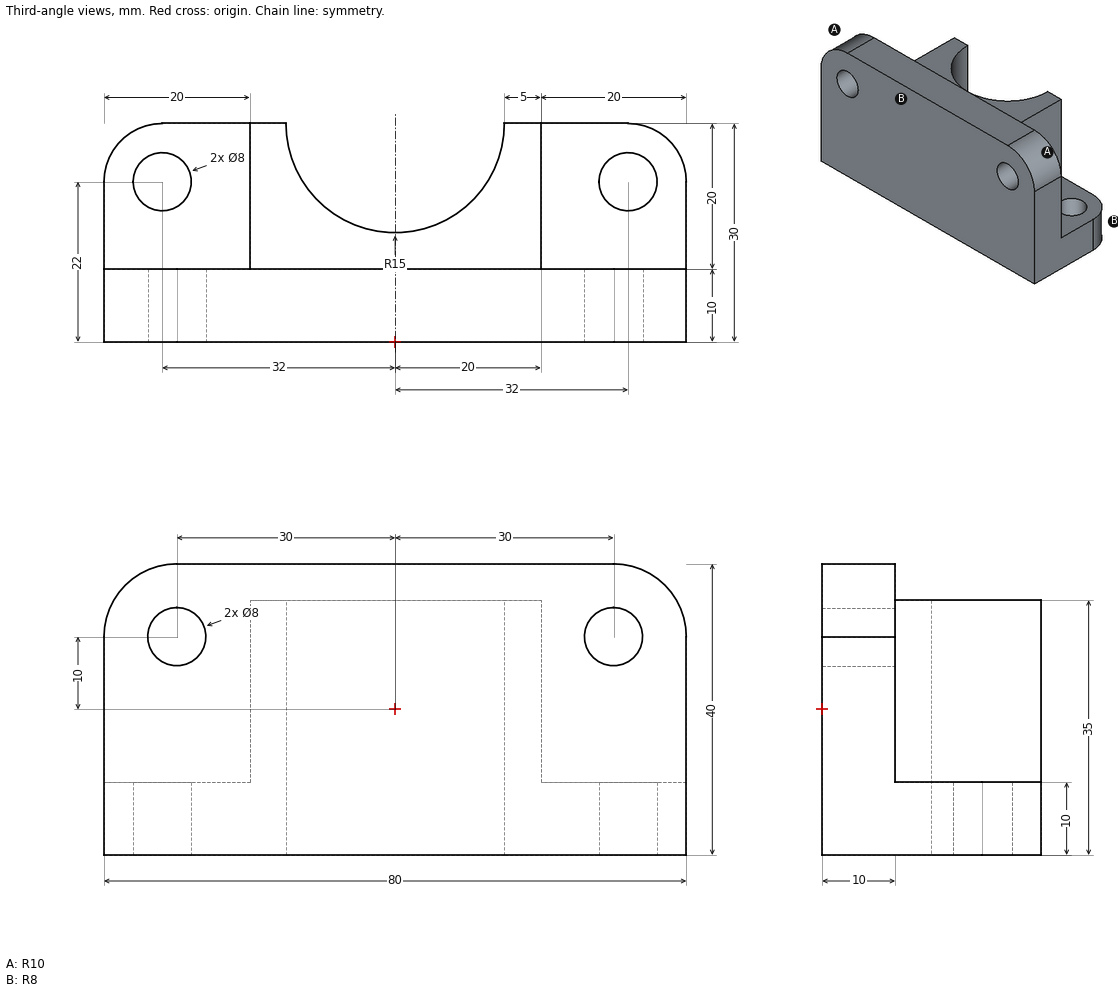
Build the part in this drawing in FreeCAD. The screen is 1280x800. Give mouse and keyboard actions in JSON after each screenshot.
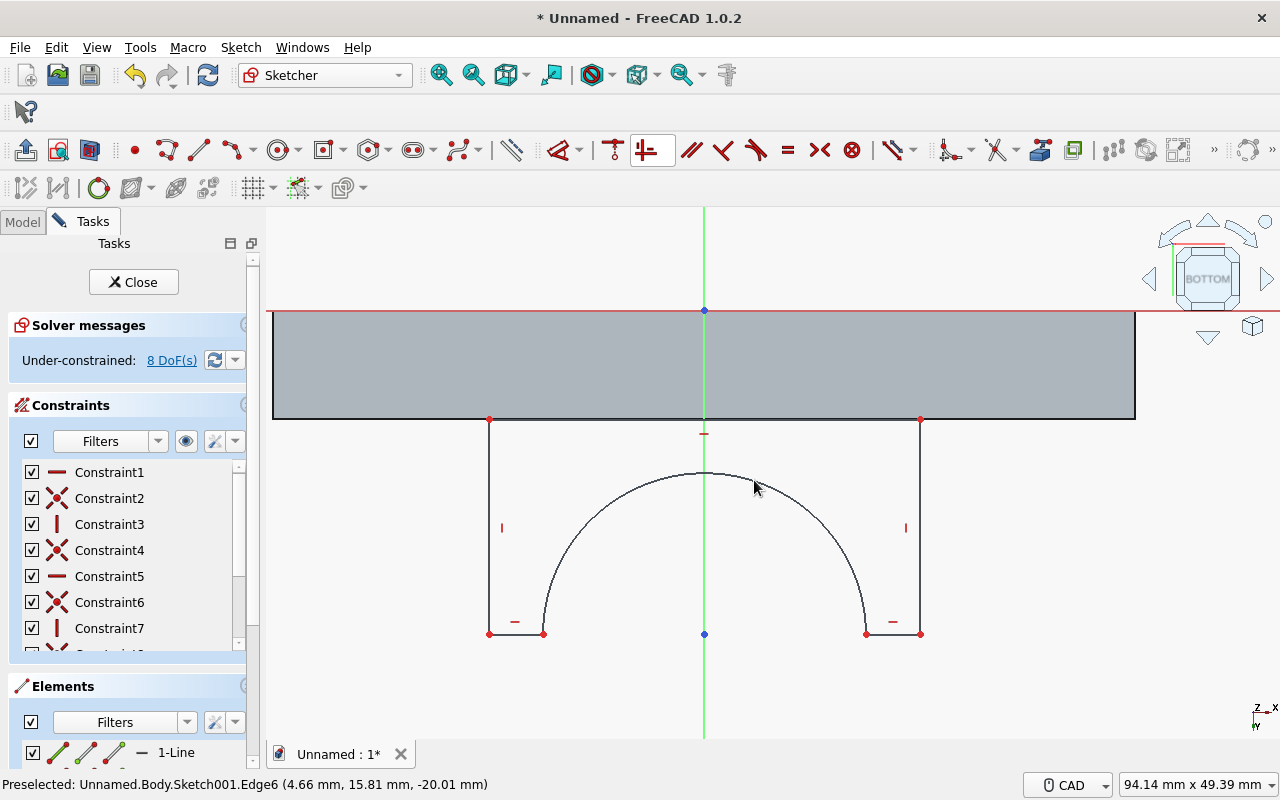
{"action": "left_click", "coordinate": [705, 635]}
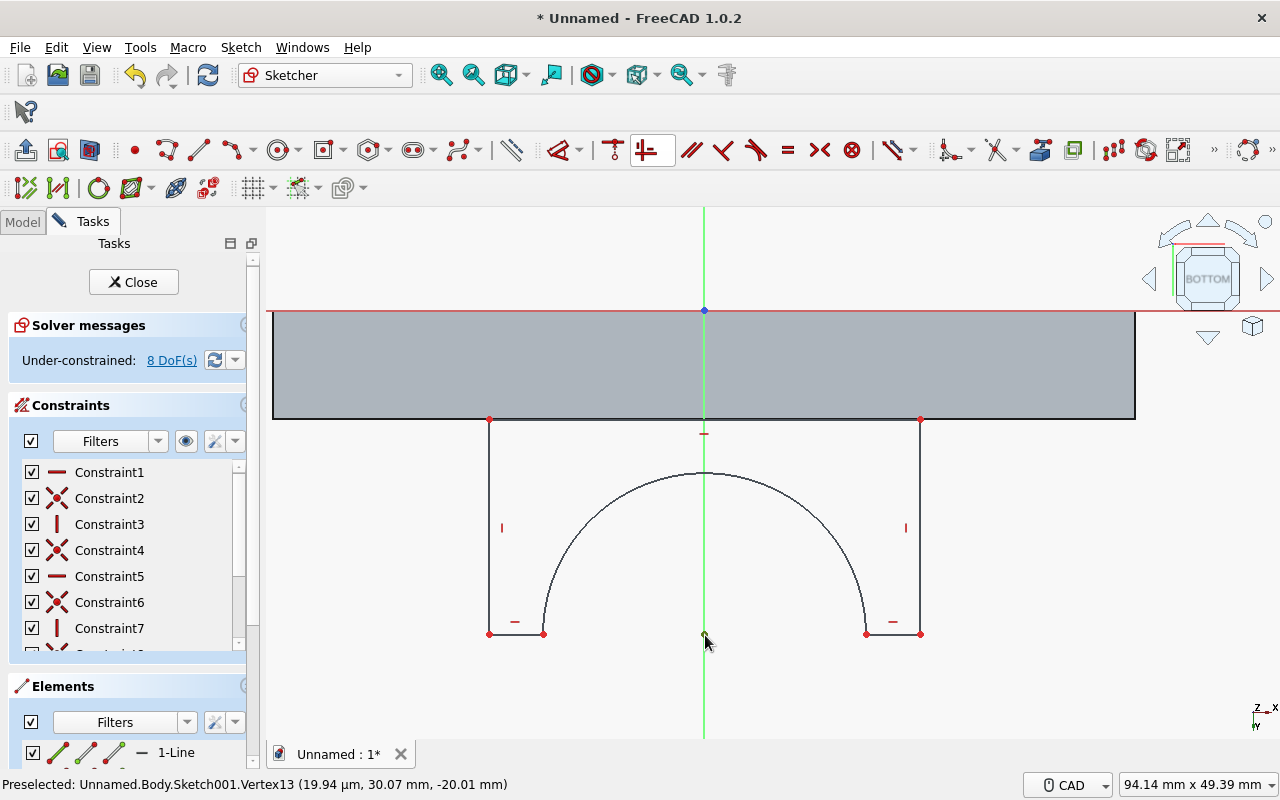
{"action": "left_click", "coordinate": [704, 677]}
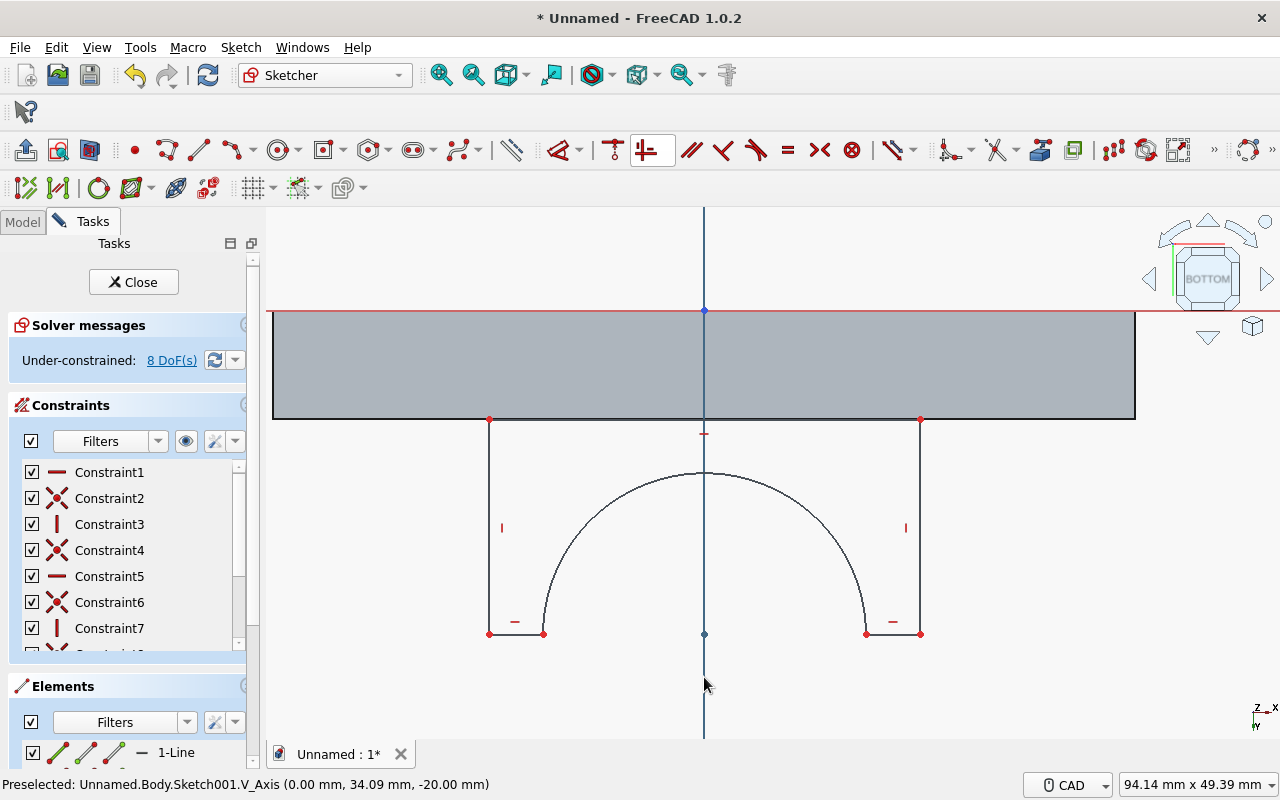
{"action": "left_click", "coordinate": [614, 150]}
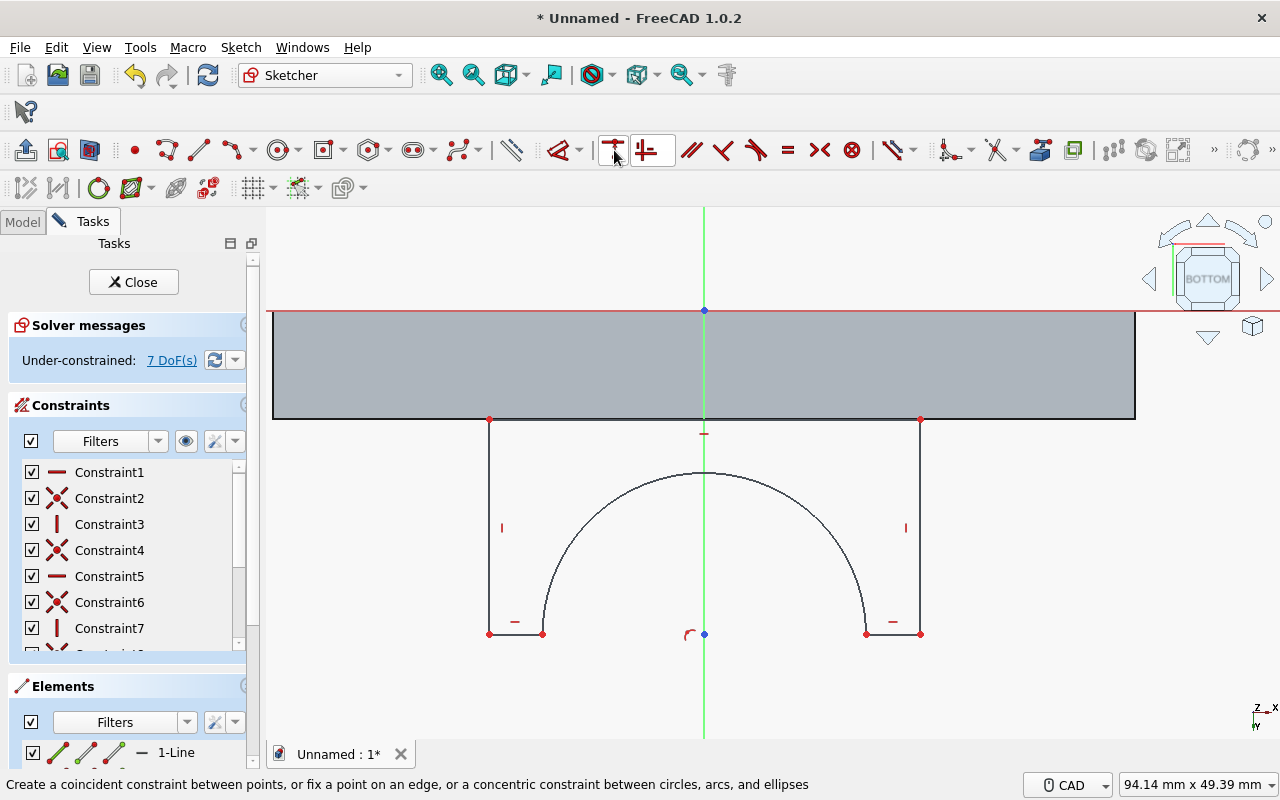
{"action": "left_click", "coordinate": [920, 635]}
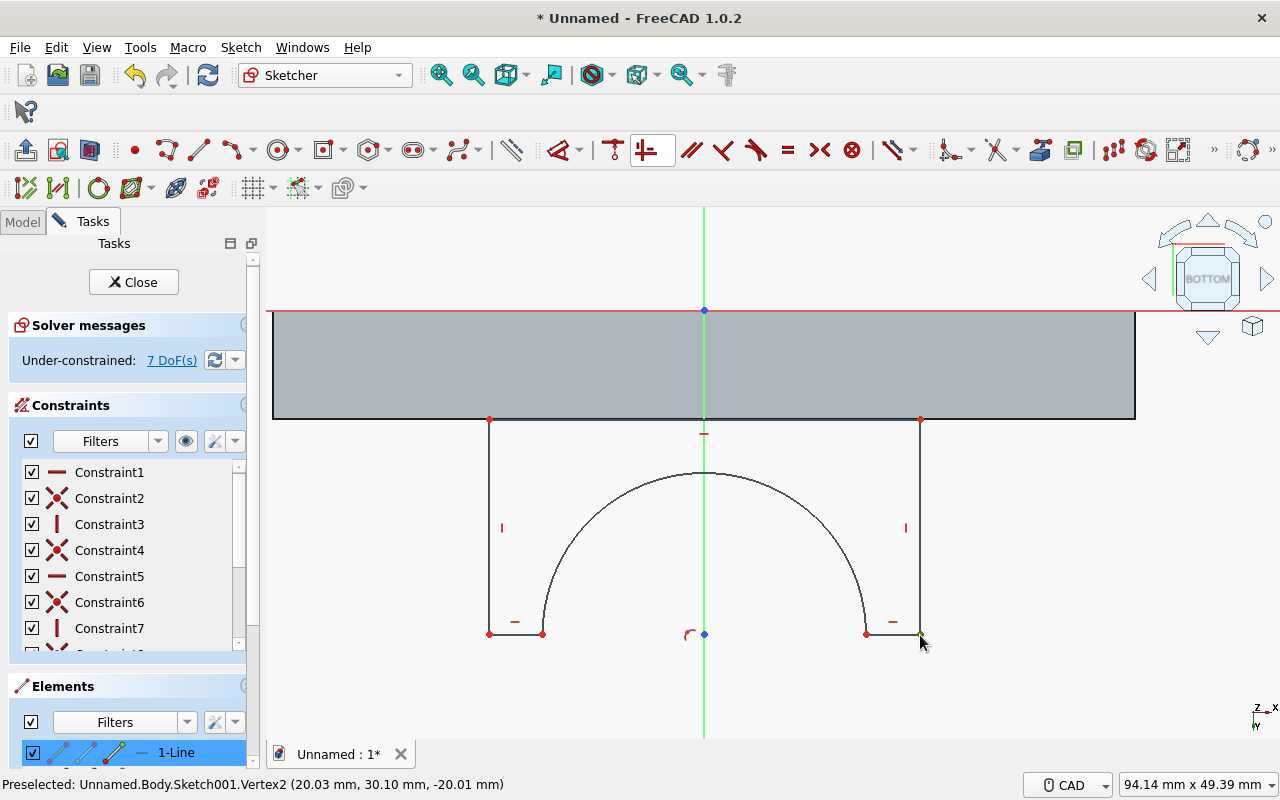
{"action": "left_click", "coordinate": [489, 635]}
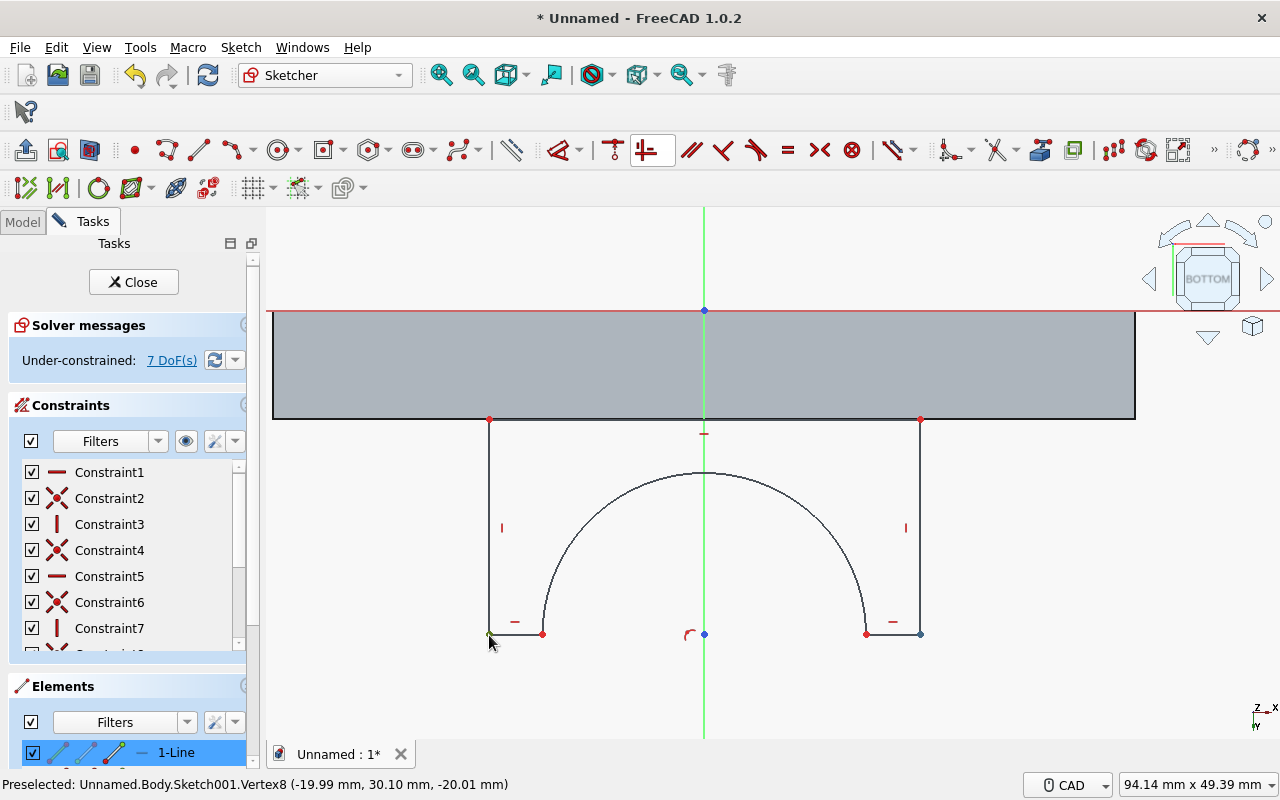
{"action": "left_click", "coordinate": [704, 677]}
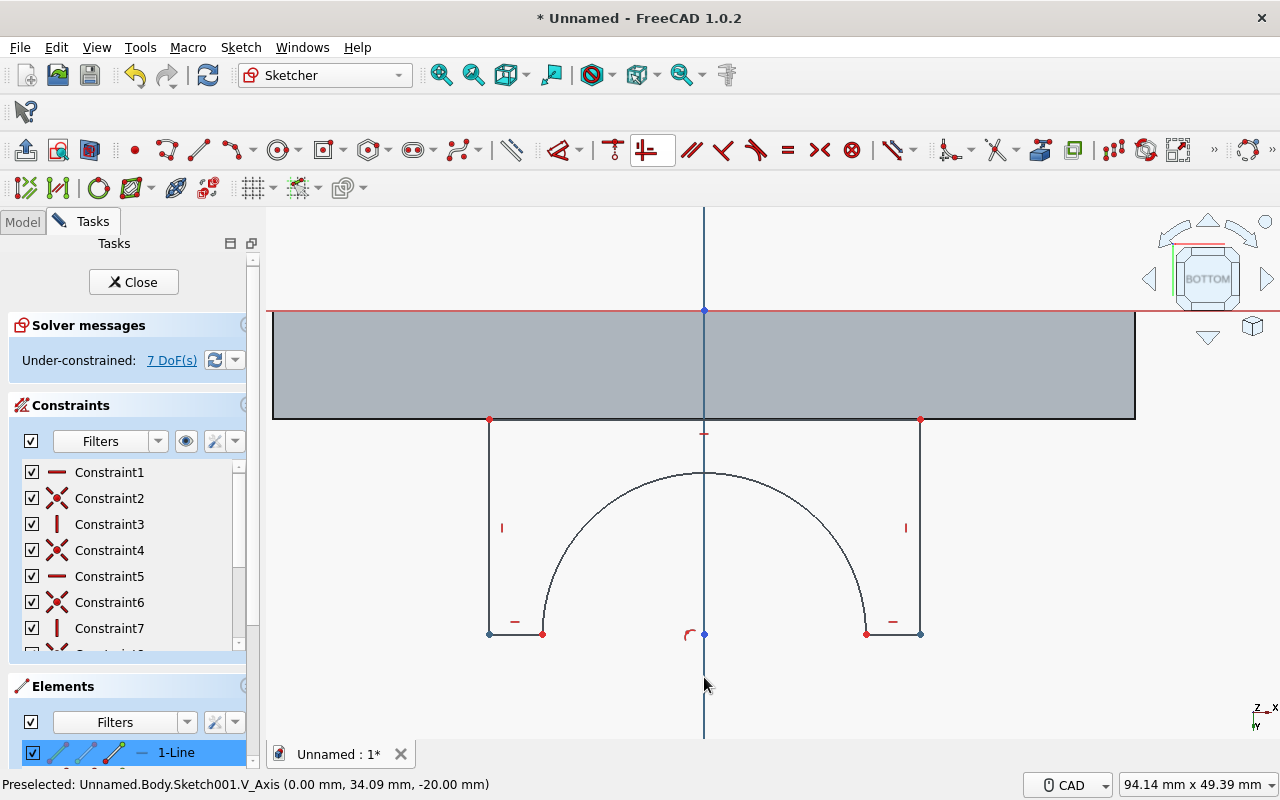
{"action": "left_click", "coordinate": [820, 150]}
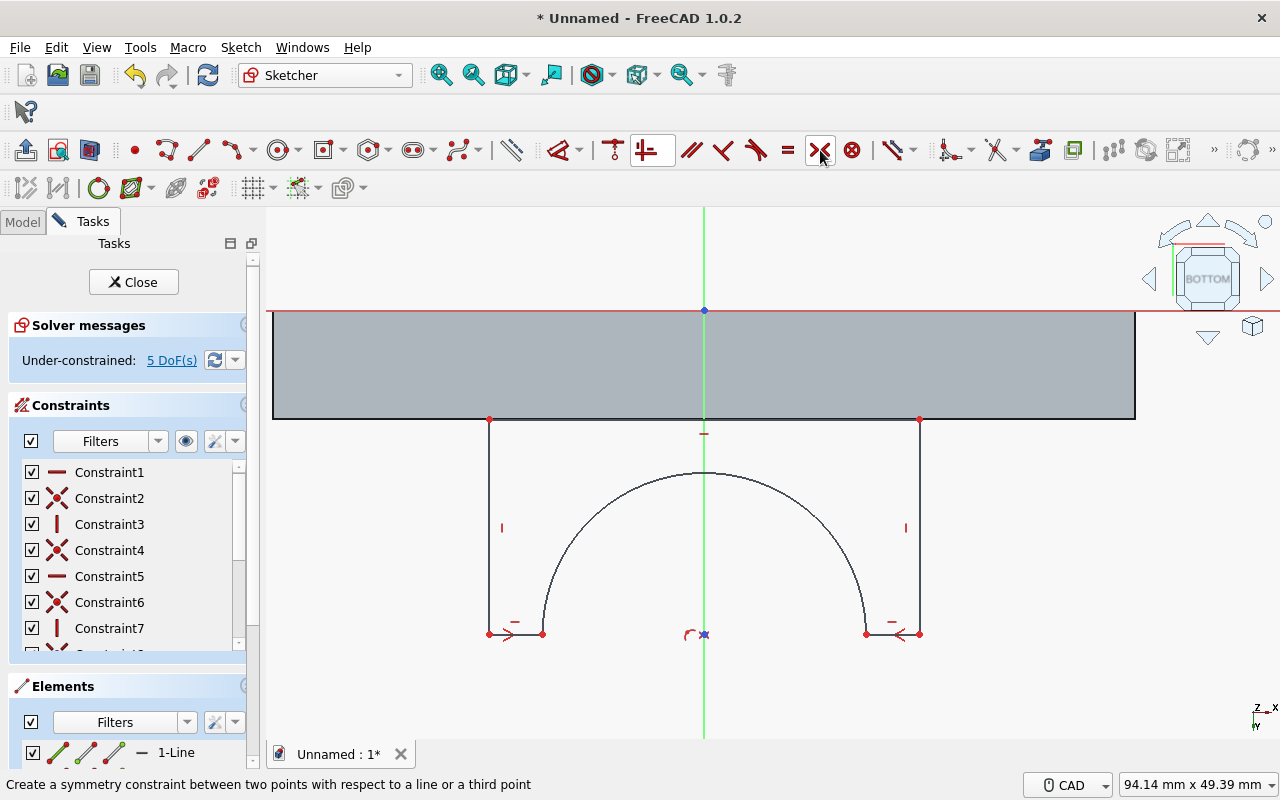
{"action": "left_click", "coordinate": [799, 504]}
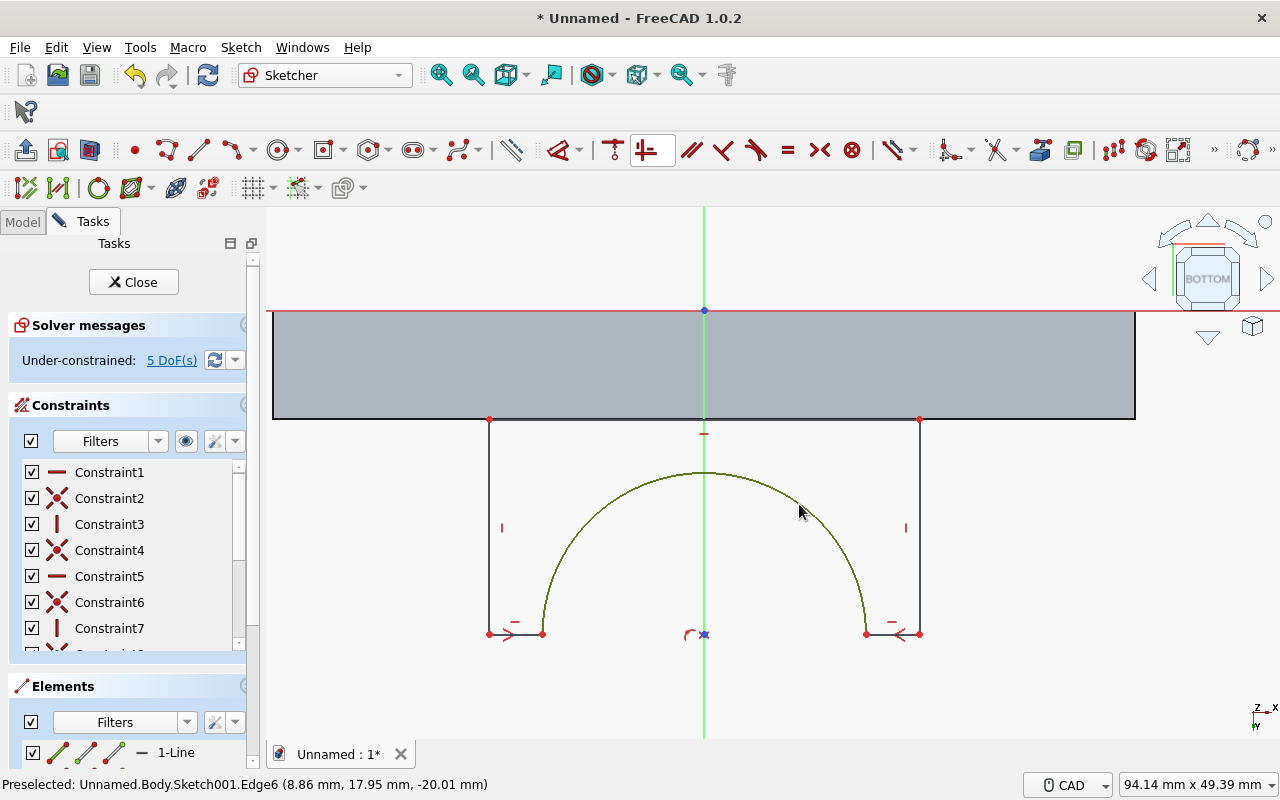
{"action": "left_click", "coordinate": [582, 150]}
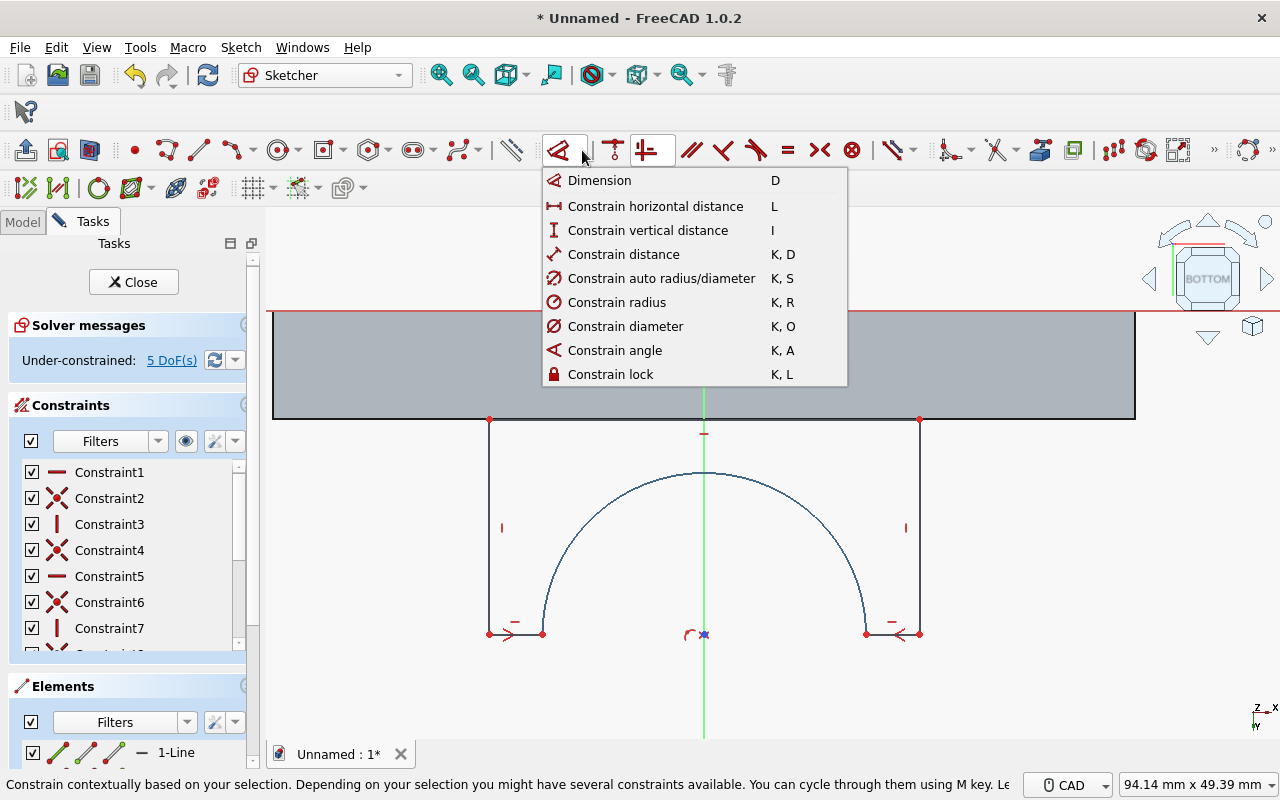
{"action": "left_click", "coordinate": [695, 302]}